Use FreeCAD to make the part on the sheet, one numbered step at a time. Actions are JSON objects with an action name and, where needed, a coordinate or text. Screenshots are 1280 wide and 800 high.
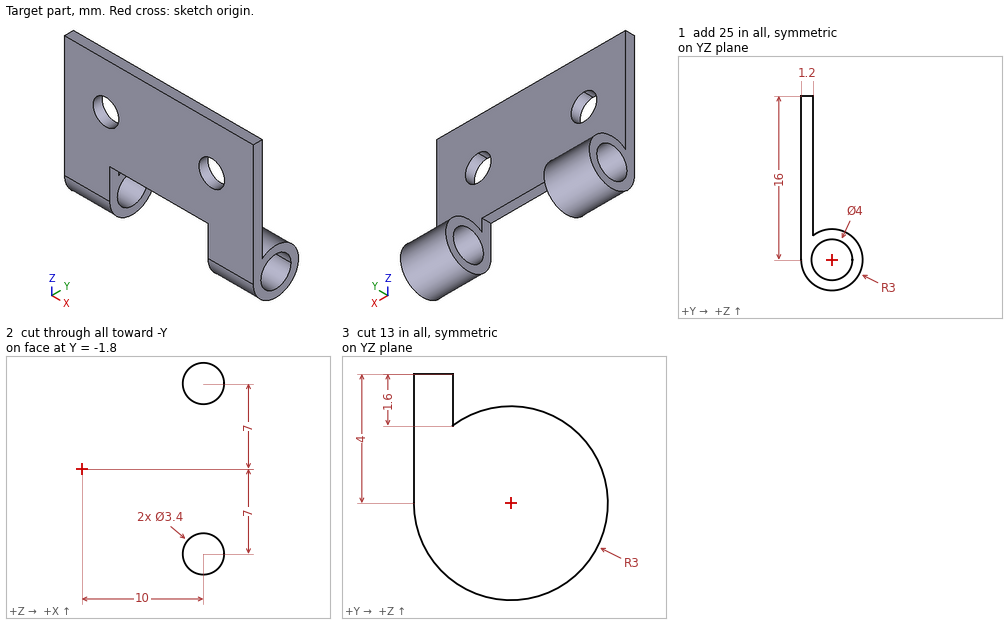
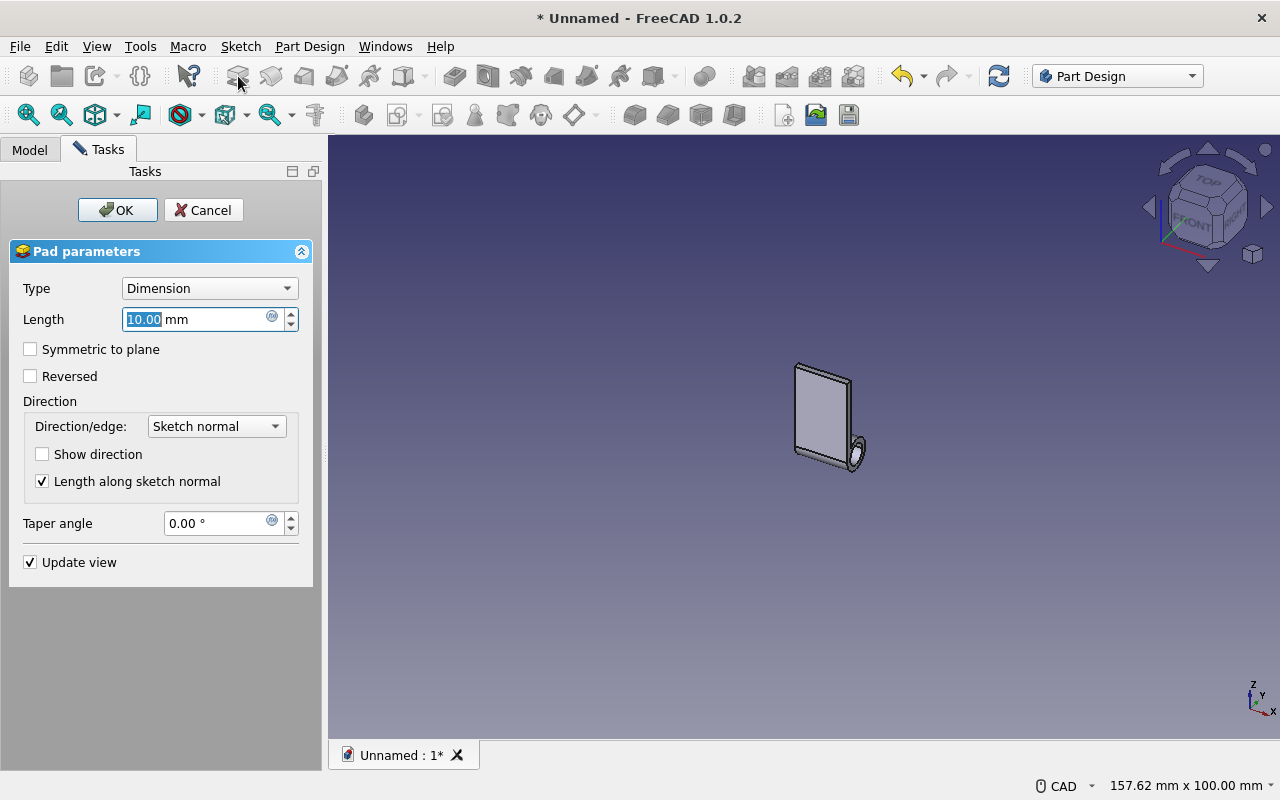
{"action": "type", "text": "25"}
{"action": "key", "text": "Tab"}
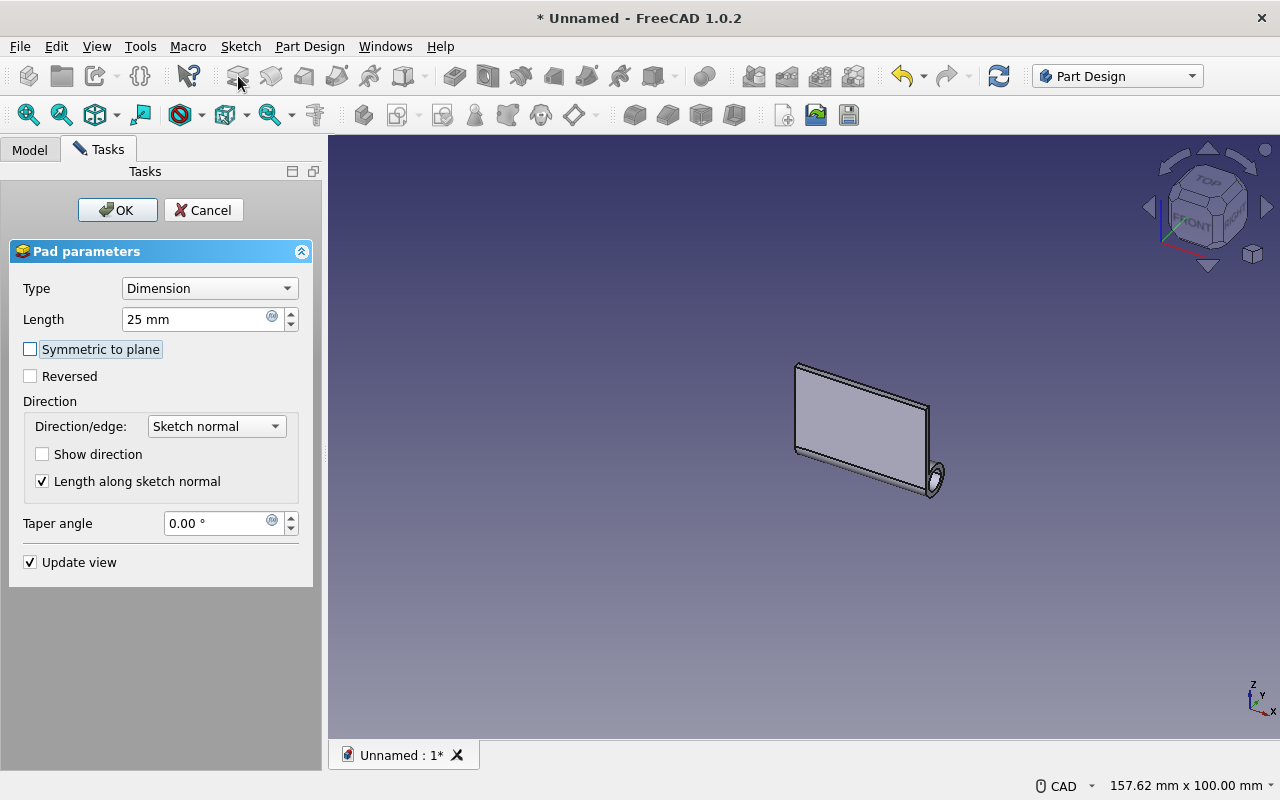
{"action": "left_click", "coordinate": [31, 349]}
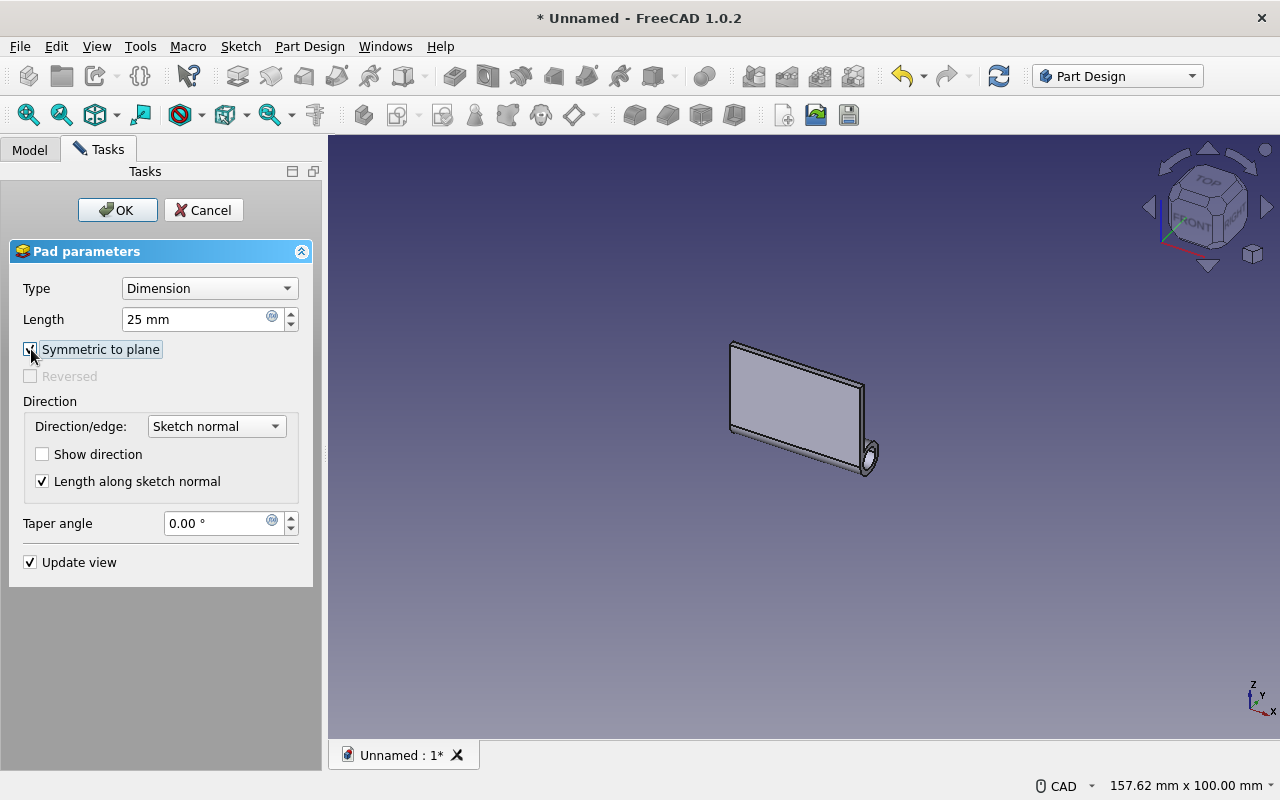
{"action": "left_click", "coordinate": [118, 210]}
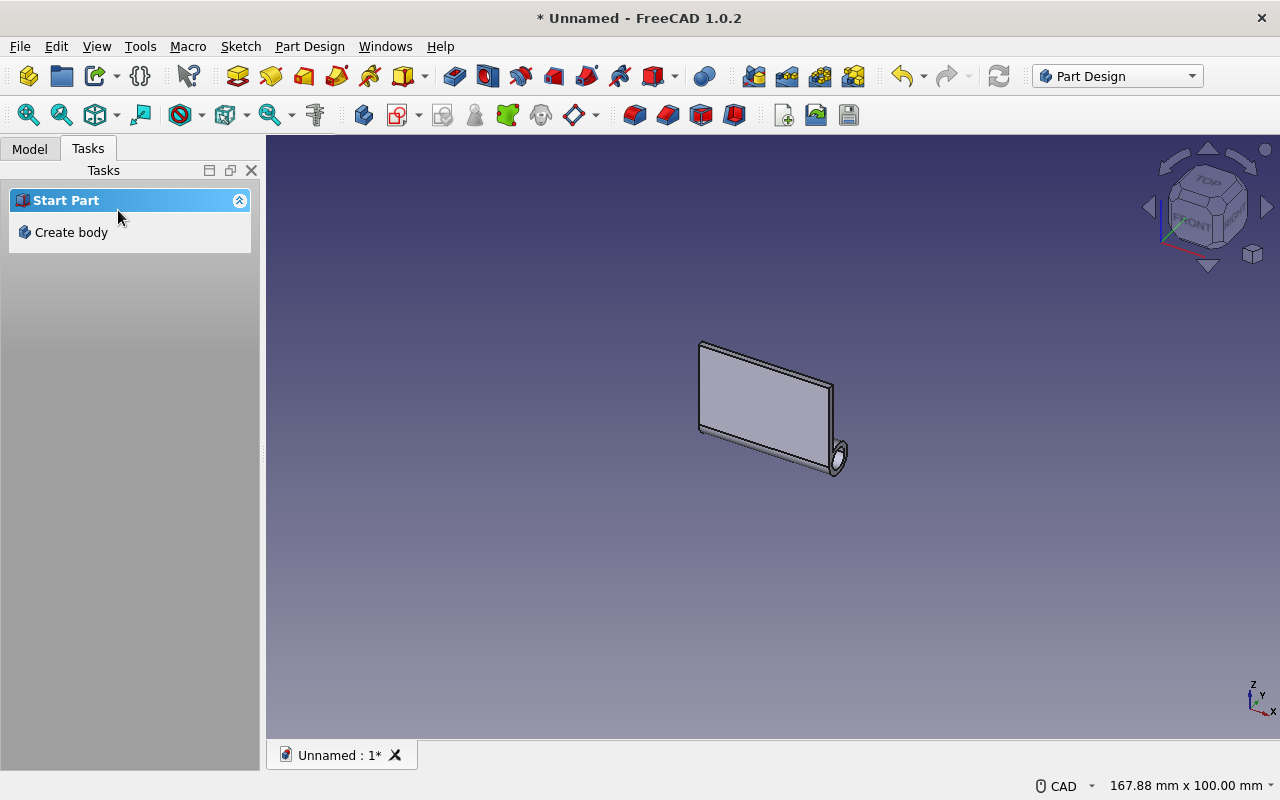
{"action": "left_click", "coordinate": [29, 116]}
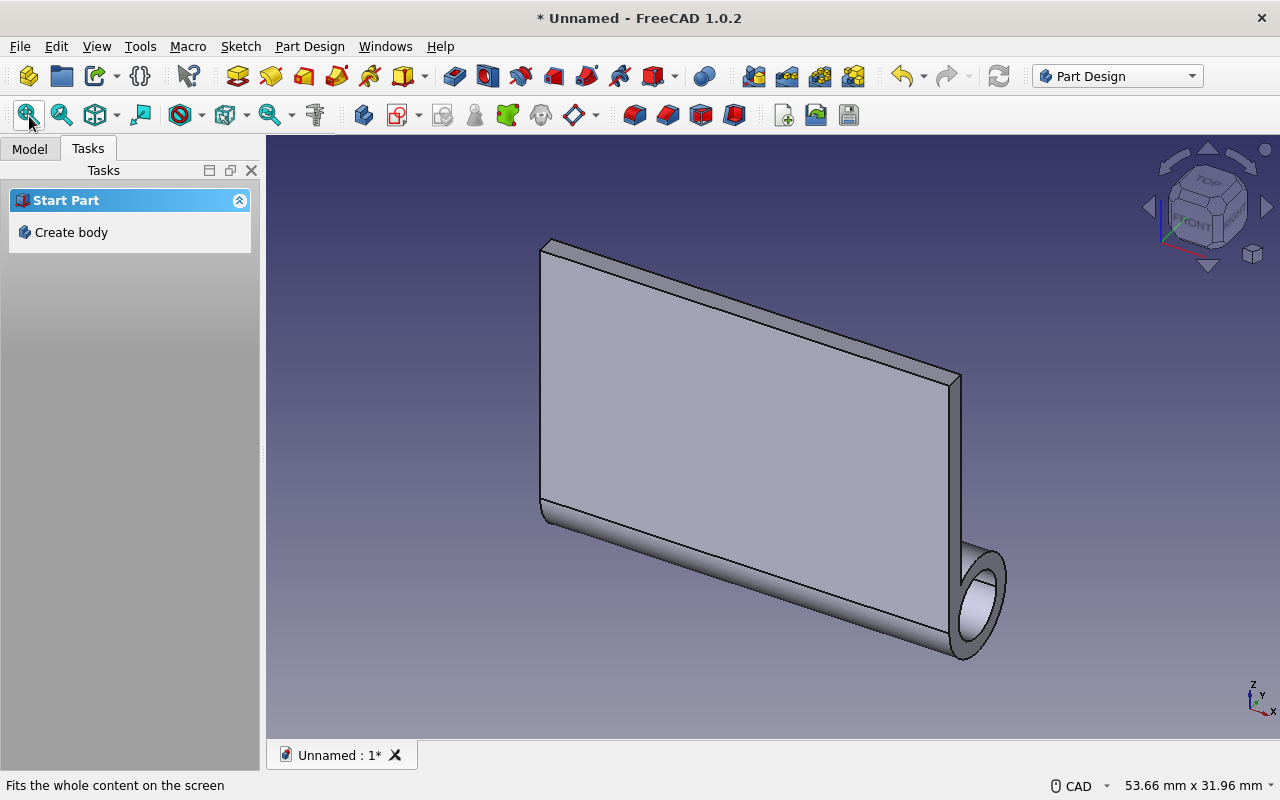
{"action": "key", "text": "4"}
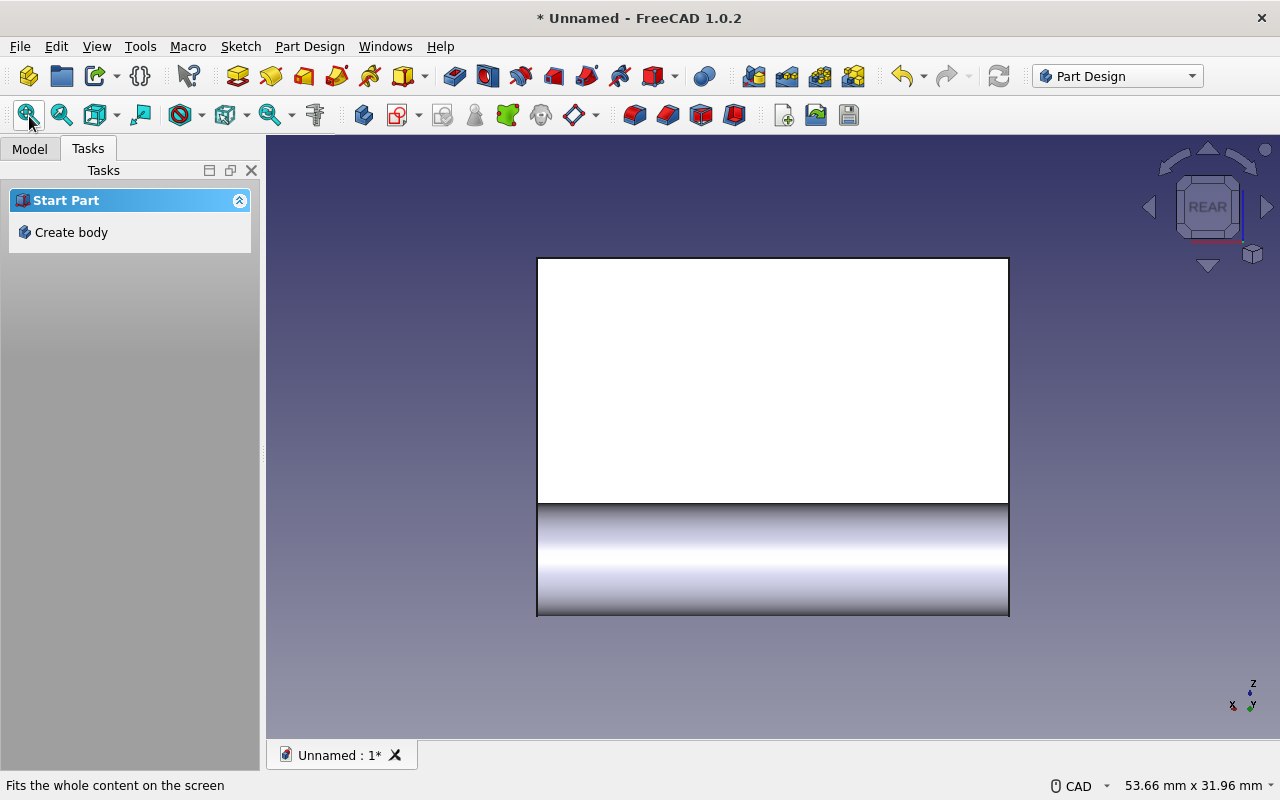
{"action": "left_click", "coordinate": [706, 385]}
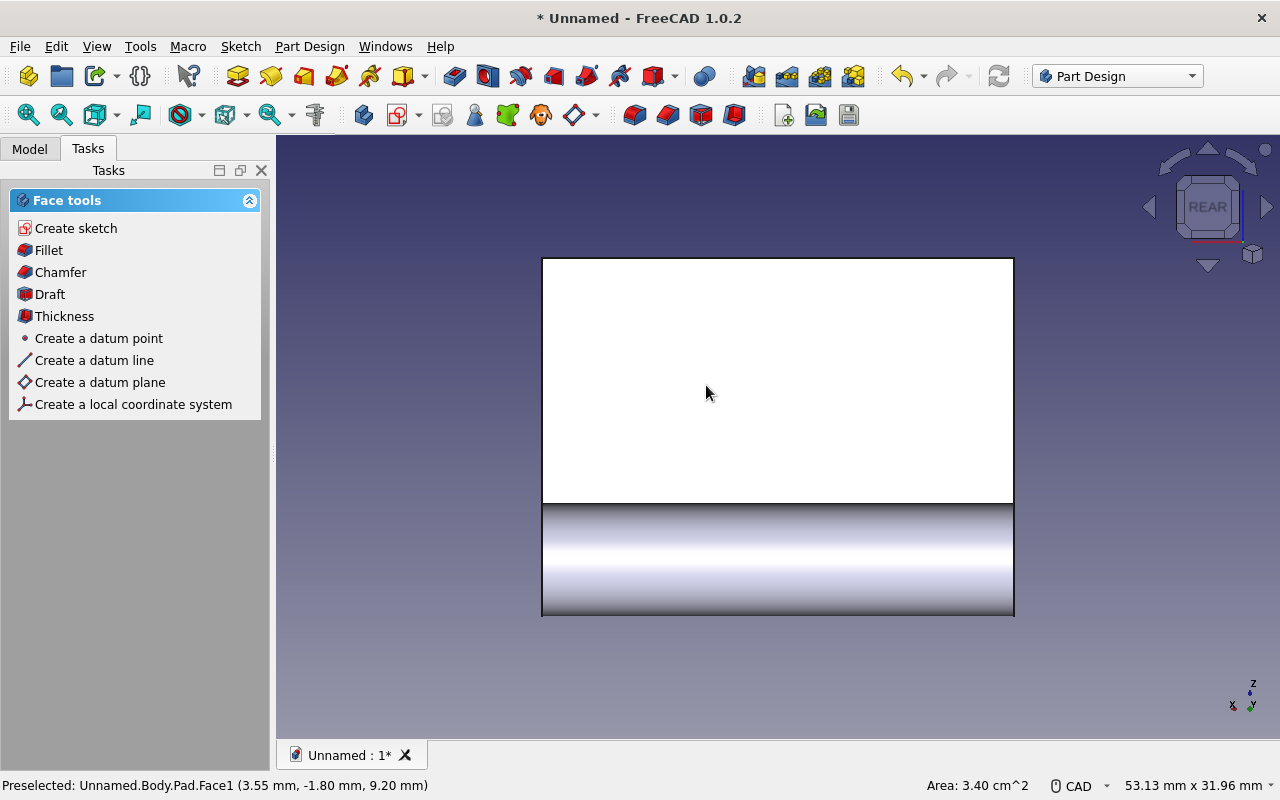
{"action": "left_click", "coordinate": [396, 116]}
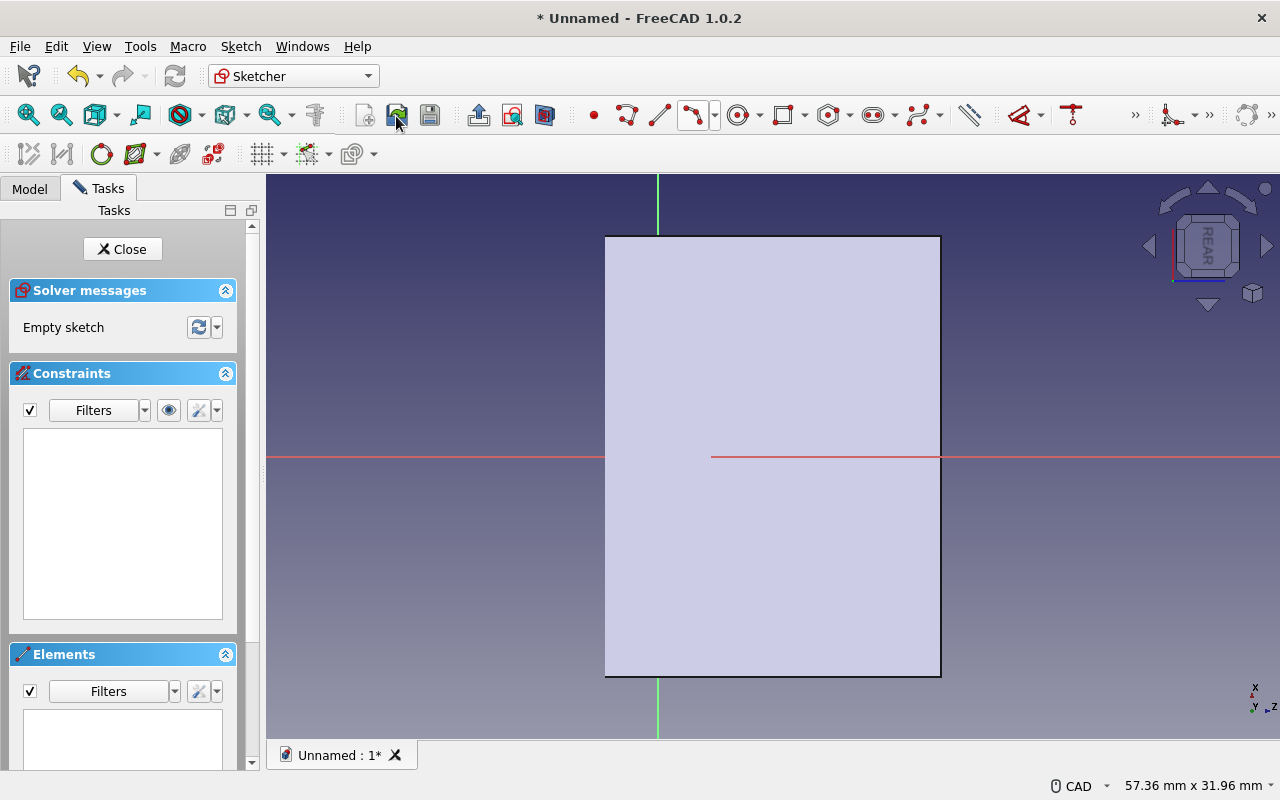
{"action": "left_click", "coordinate": [738, 116]}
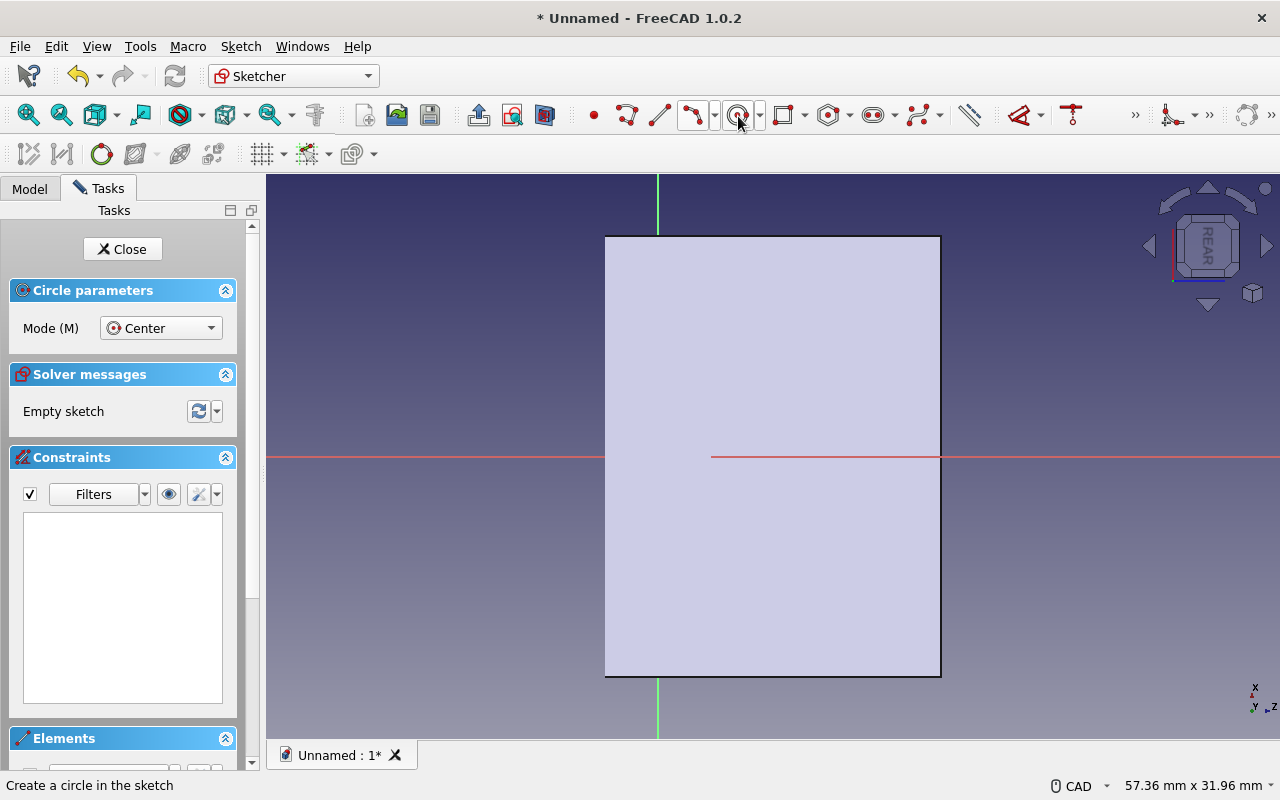
{"action": "left_click", "coordinate": [835, 580]}
{"action": "left_click", "coordinate": [856, 559]}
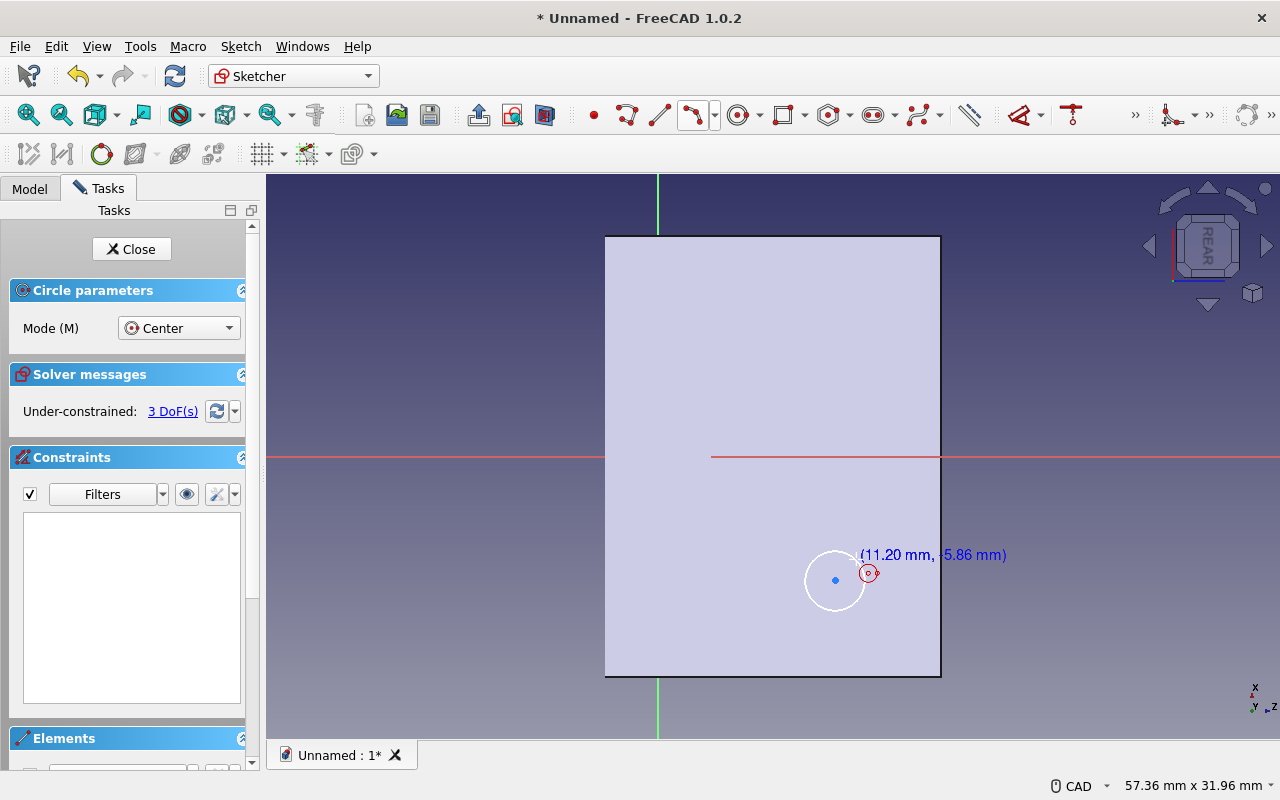
{"action": "left_click", "coordinate": [835, 333]}
{"action": "left_click", "coordinate": [856, 312]}
{"action": "key", "text": "Escape"}